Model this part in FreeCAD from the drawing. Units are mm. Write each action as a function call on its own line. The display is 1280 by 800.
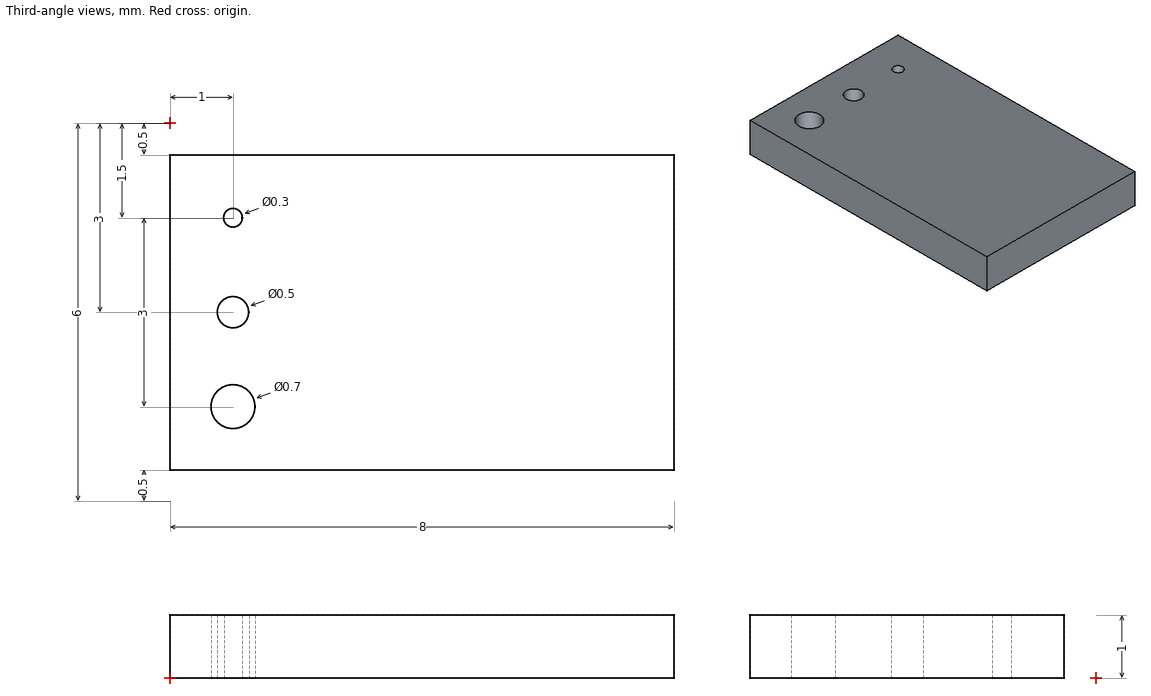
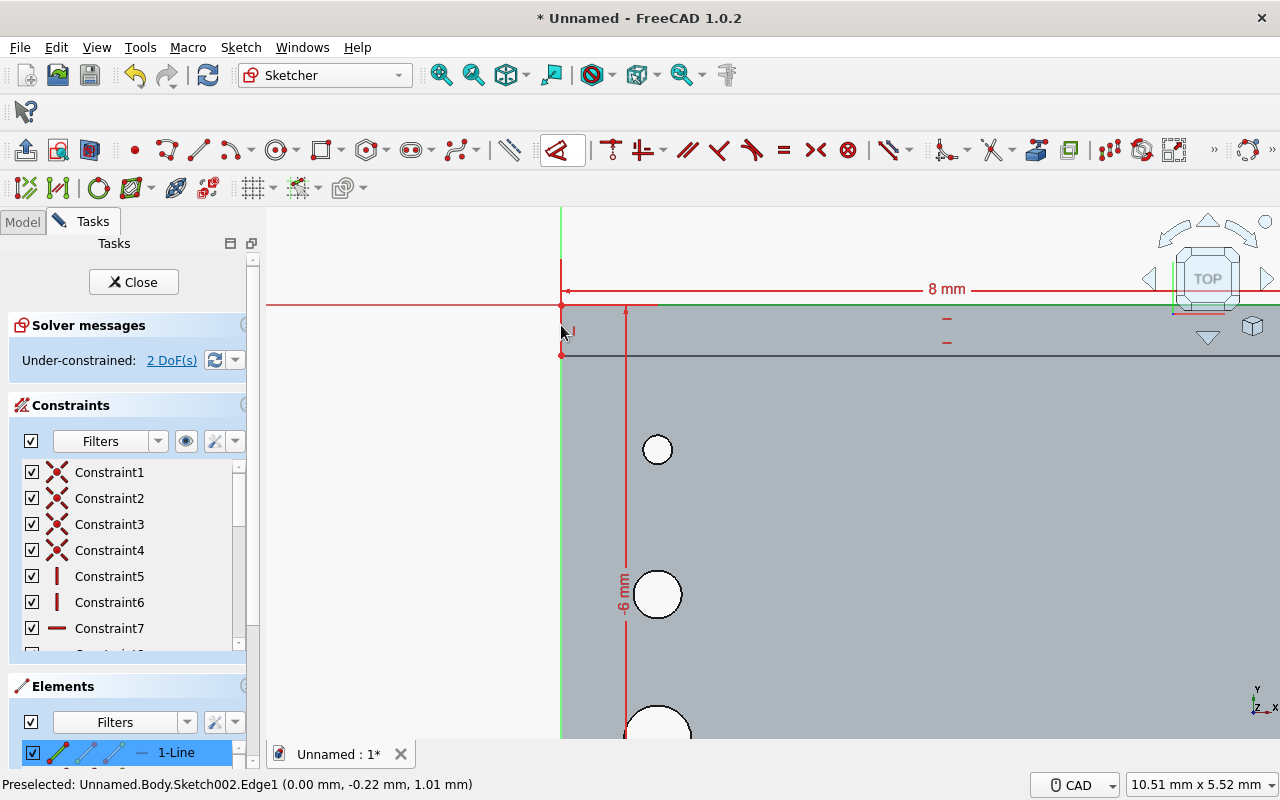
key(i)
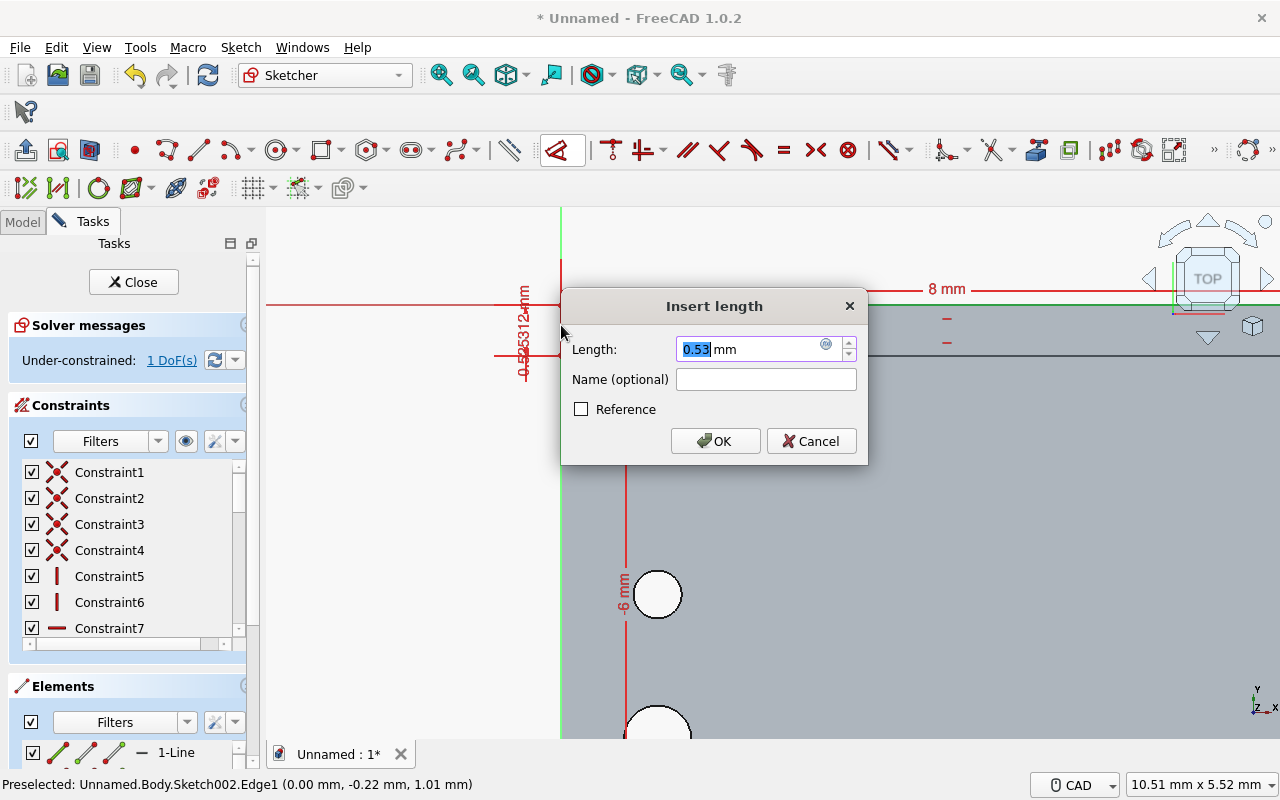
text(0.5)
key(Return)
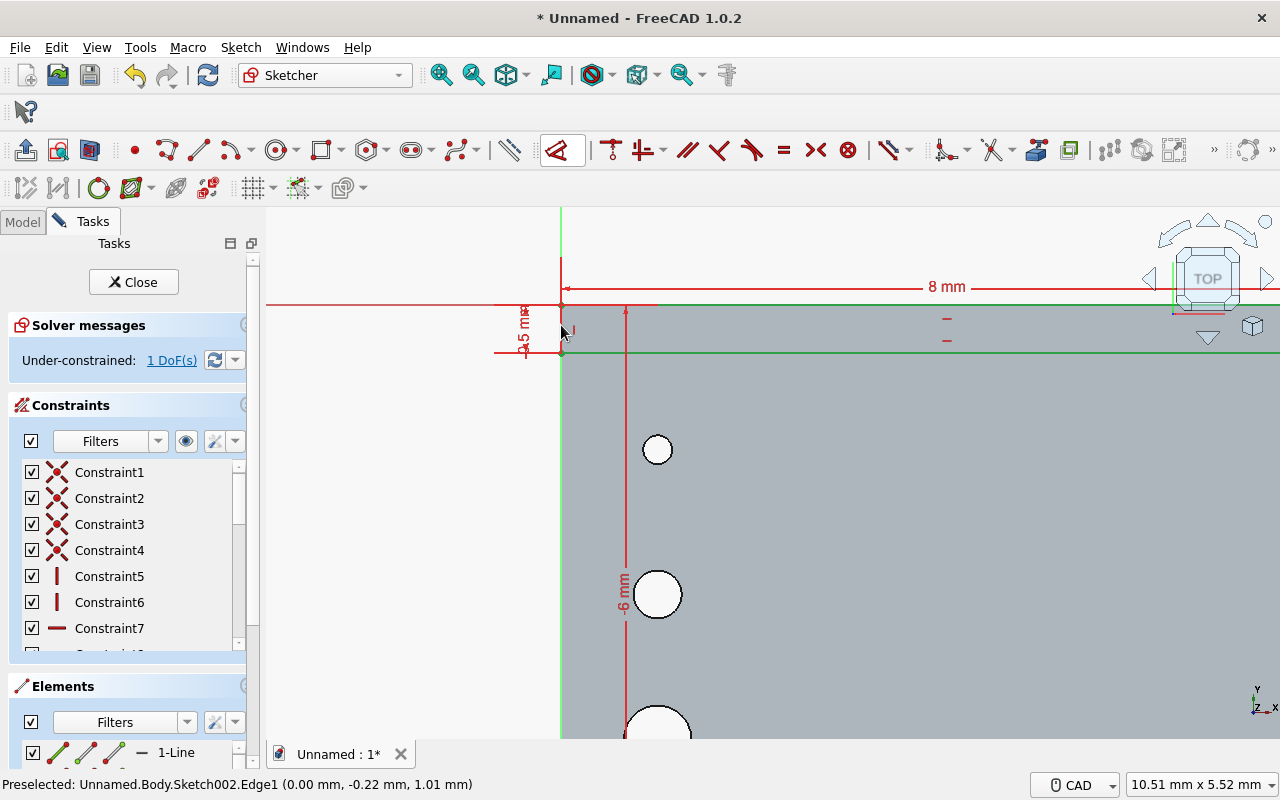
scroll(409, 325, down, 3)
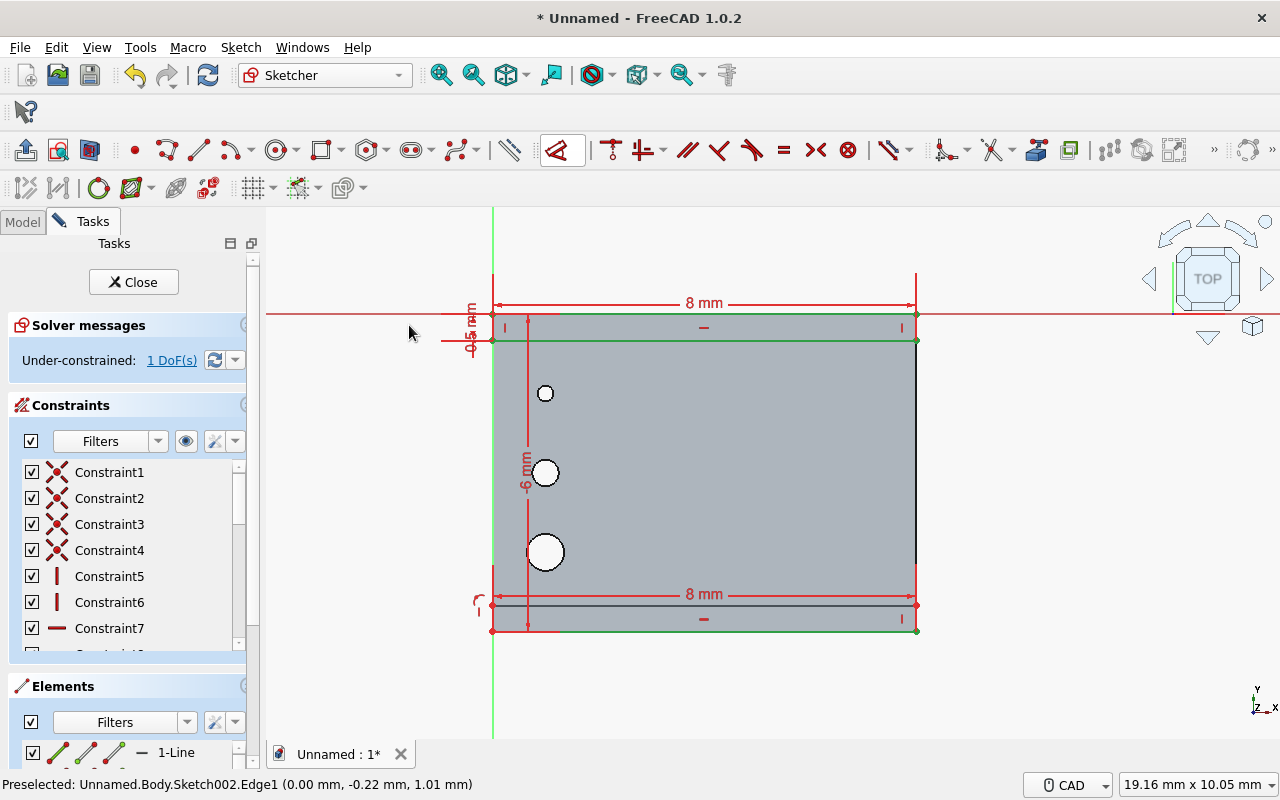
scroll(493, 614, up, 3)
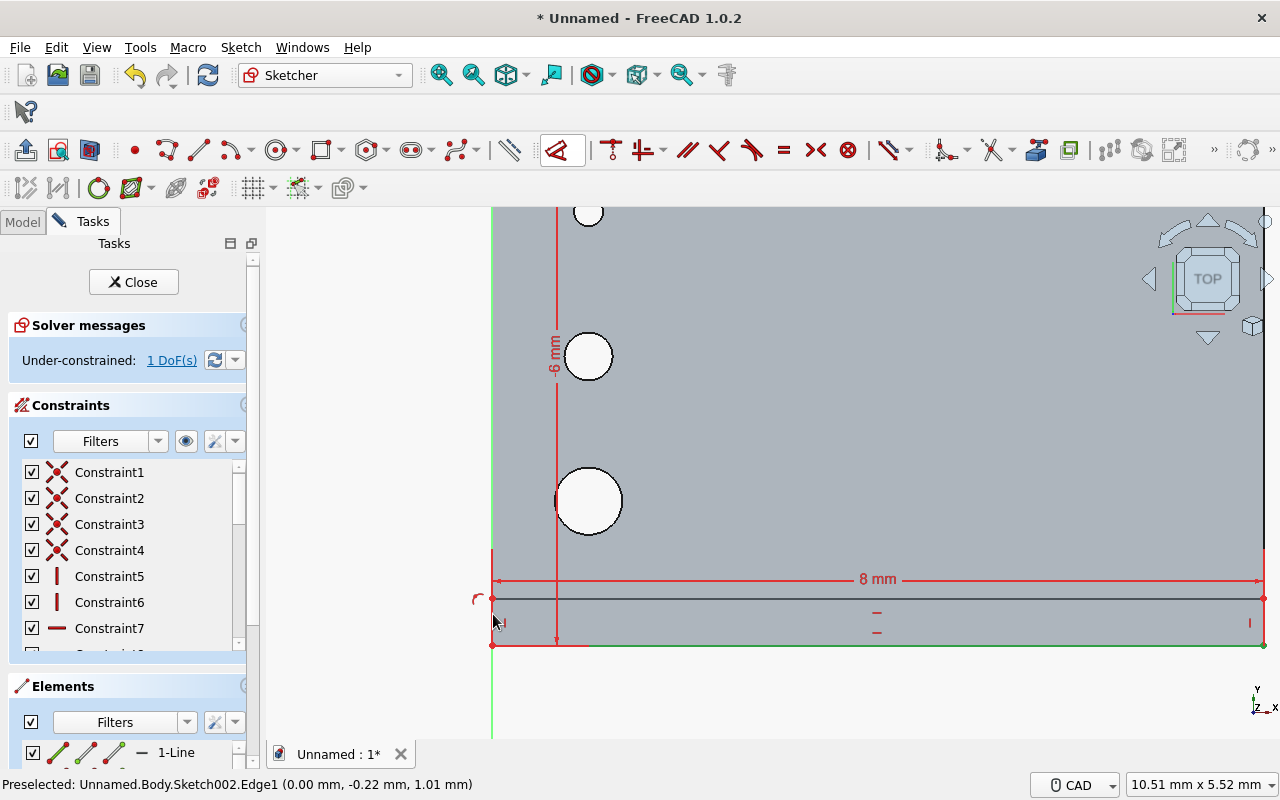
click(492, 613)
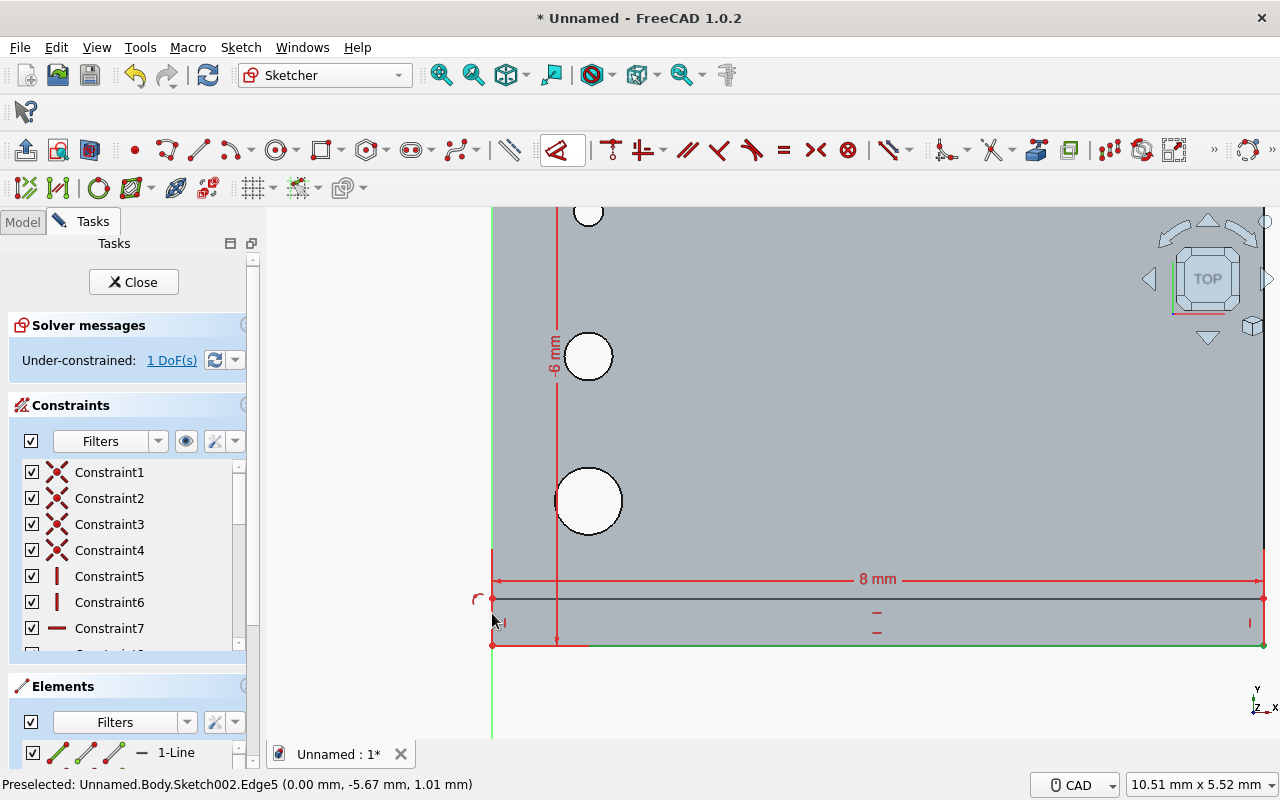
key(i)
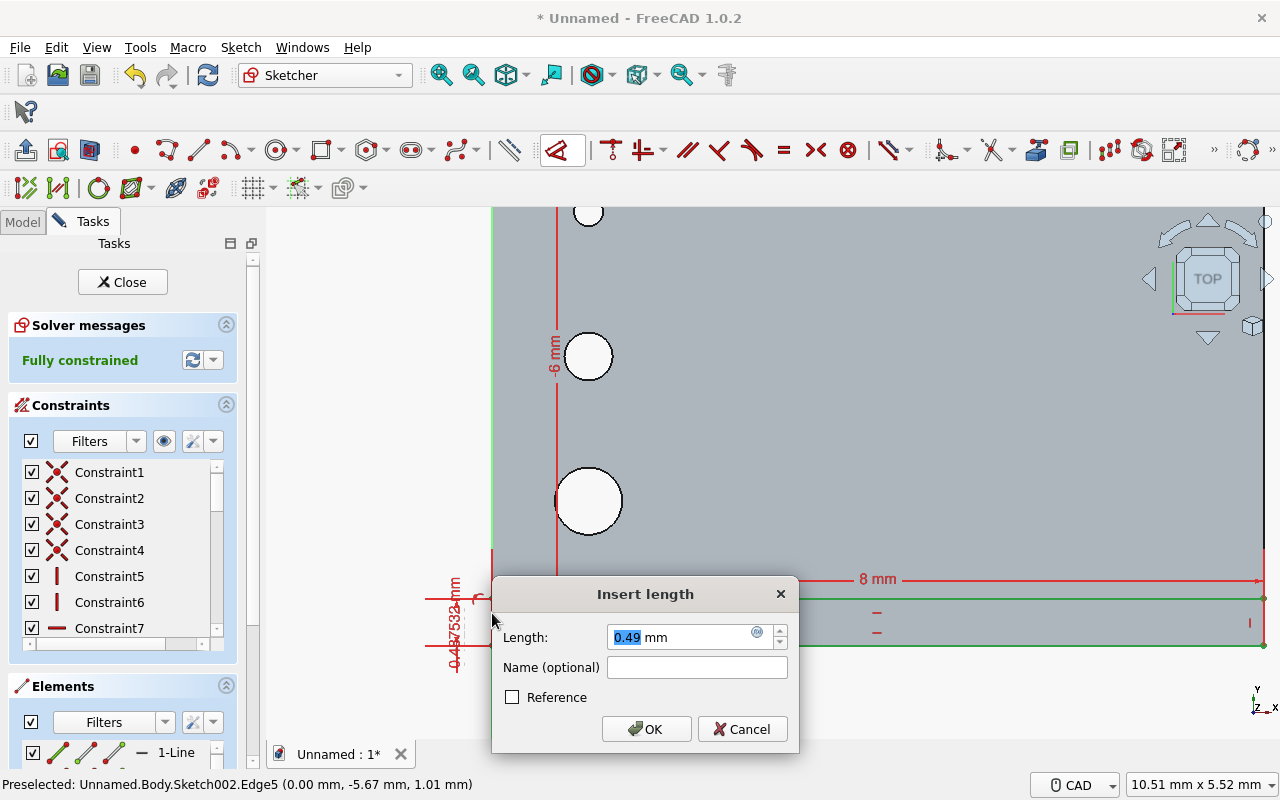
text(0.5)
key(Return)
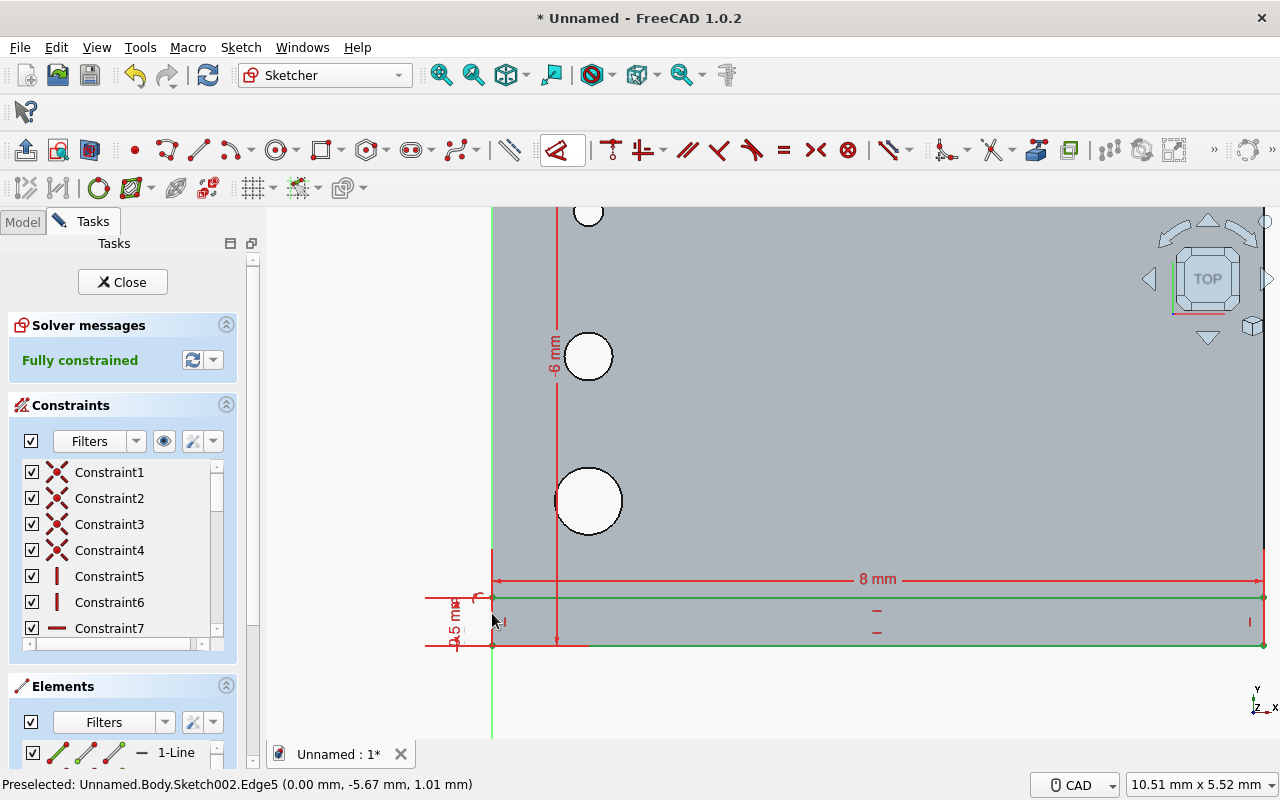
click(123, 282)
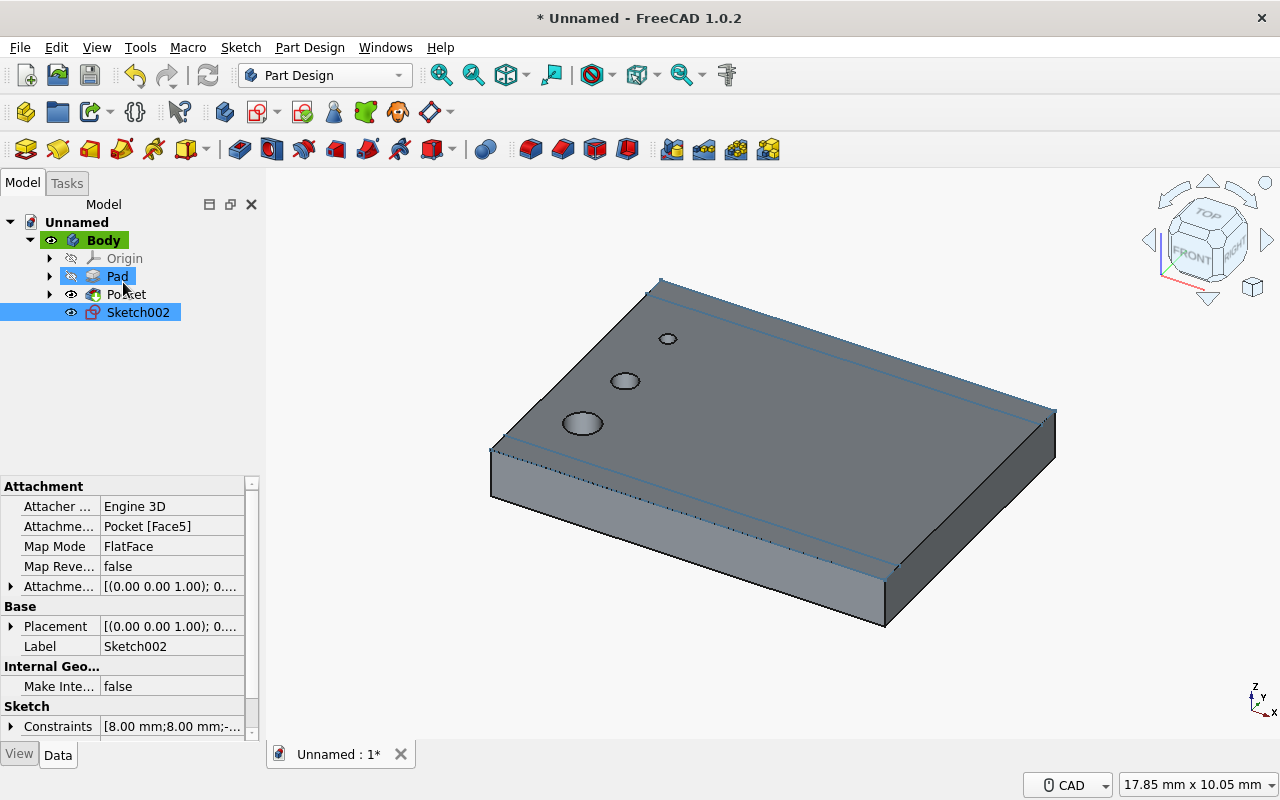
click(240, 150)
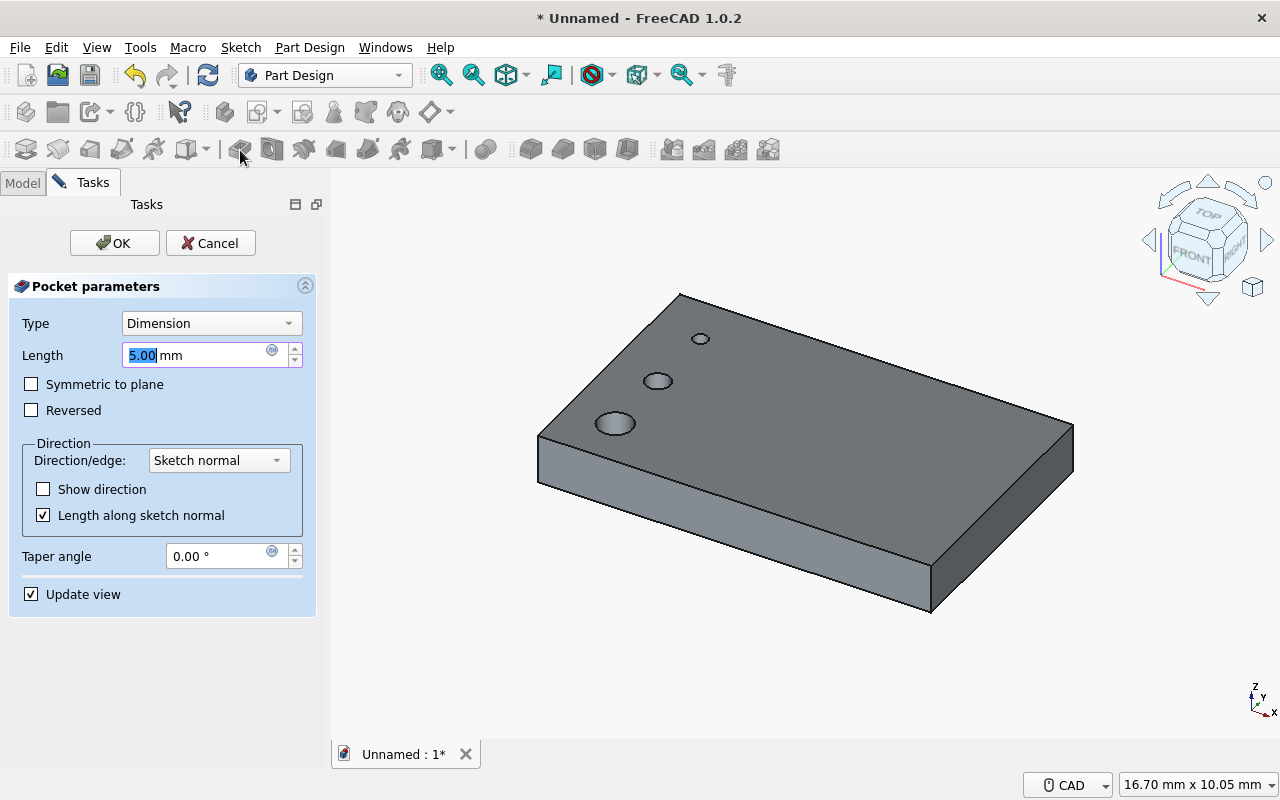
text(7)
key(Tab)